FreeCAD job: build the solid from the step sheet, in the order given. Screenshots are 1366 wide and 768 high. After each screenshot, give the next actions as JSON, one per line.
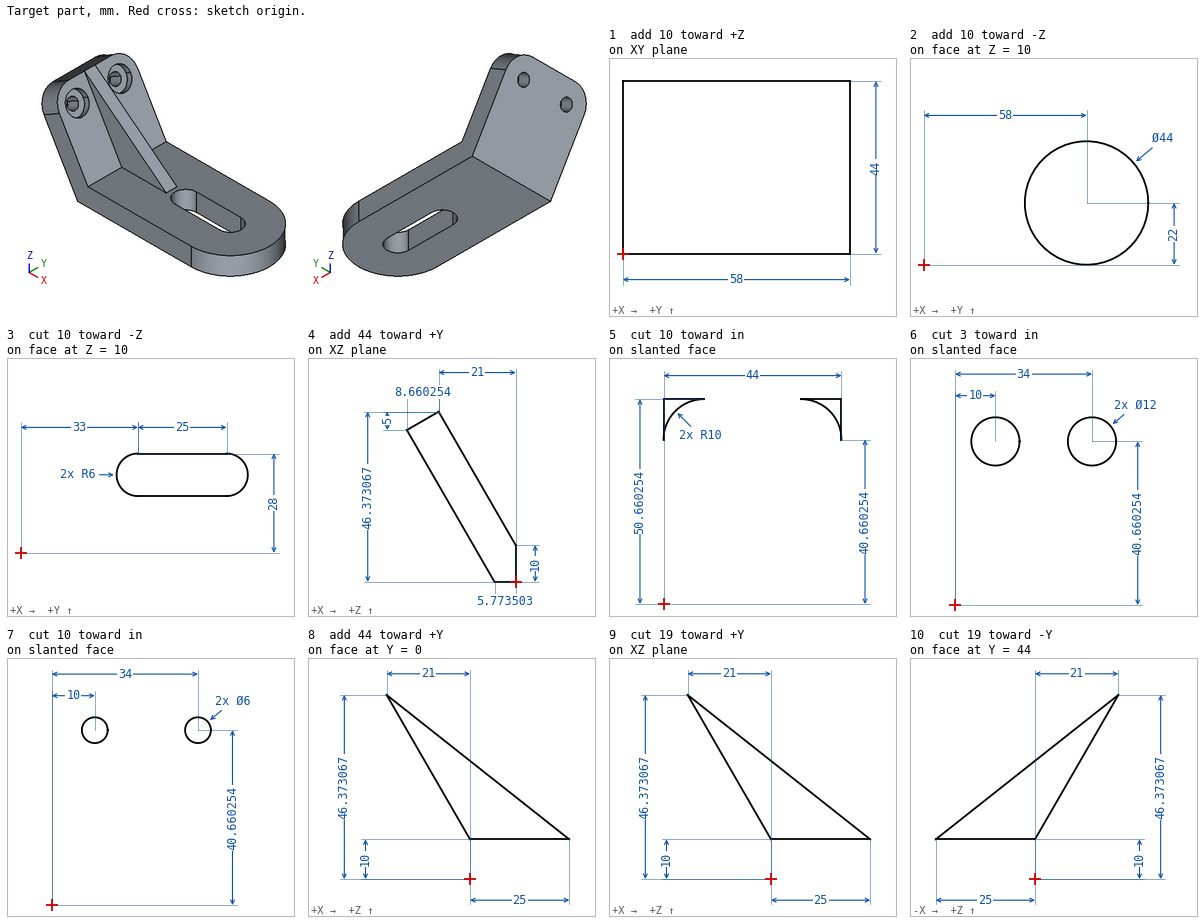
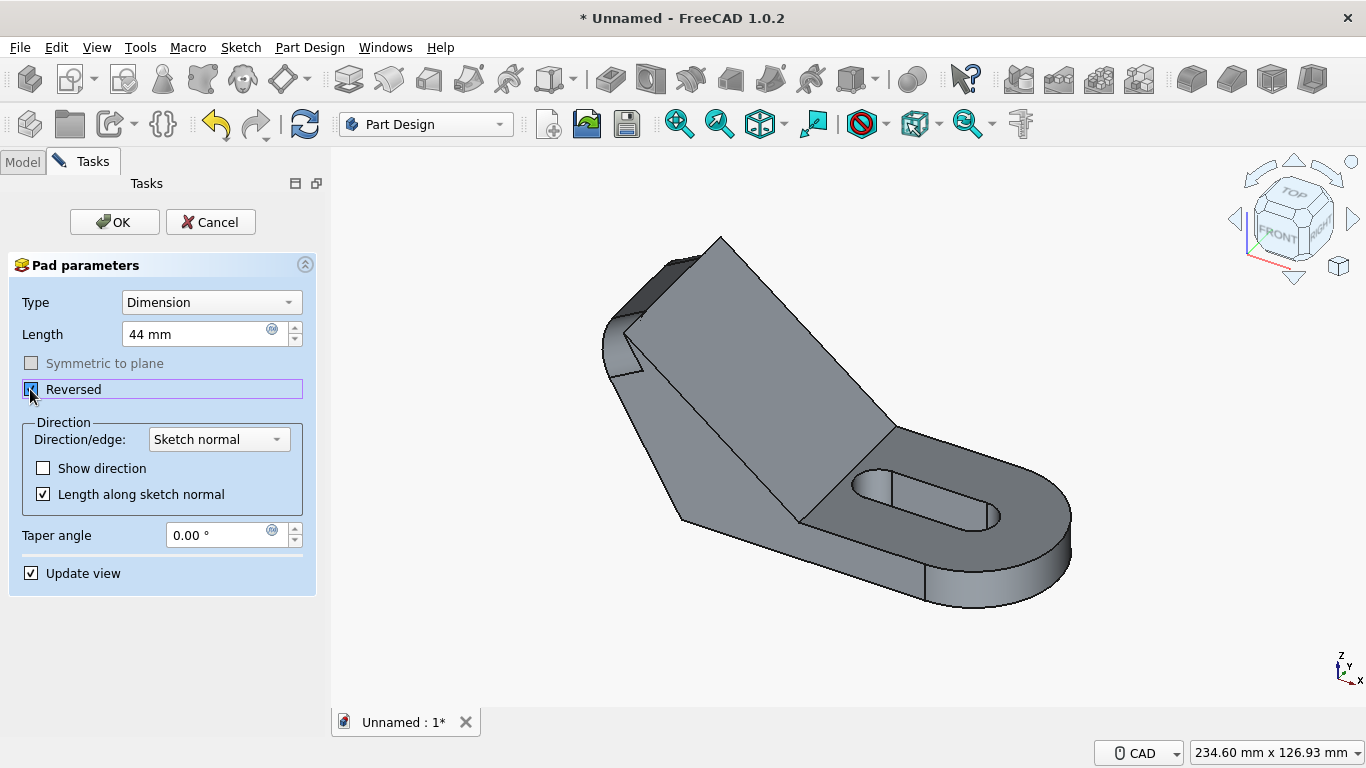
{"action": "left_click", "coordinate": [115, 222]}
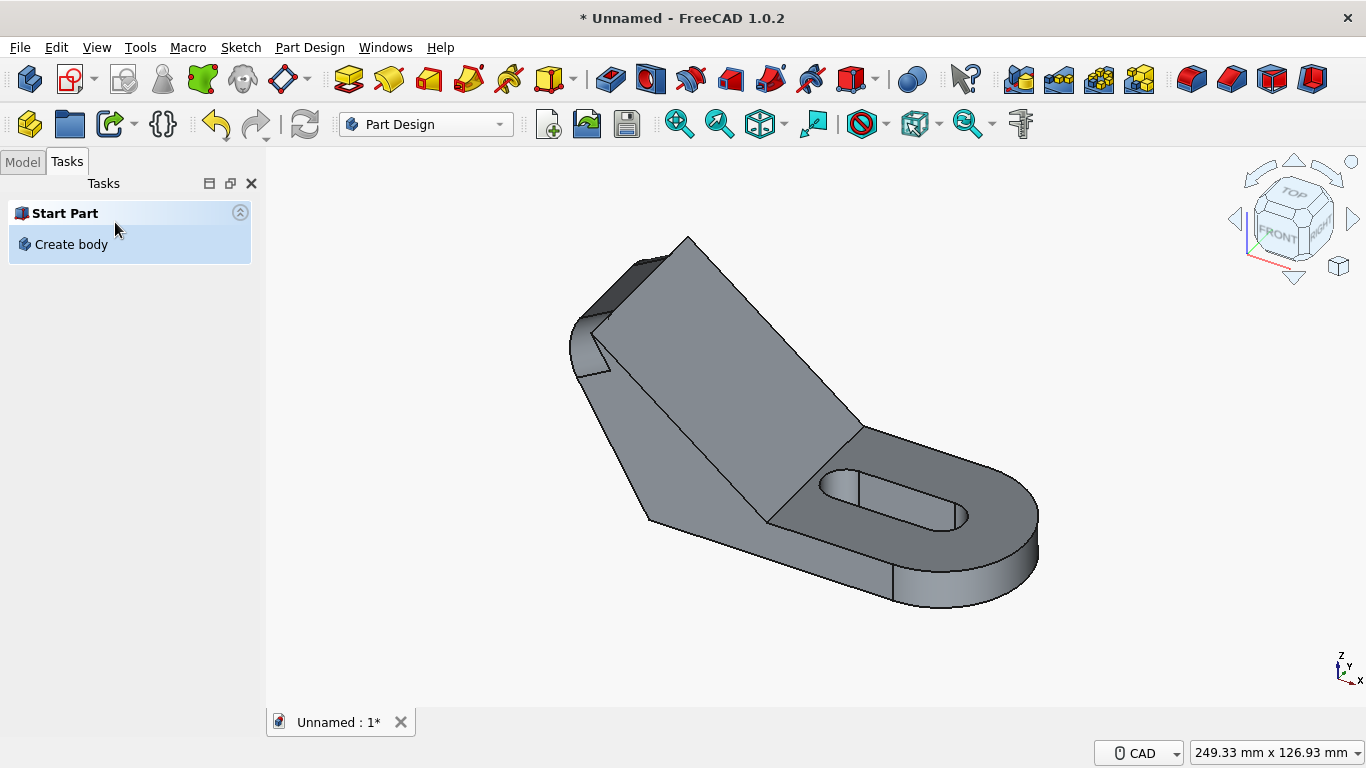
{"action": "left_click", "coordinate": [70, 80]}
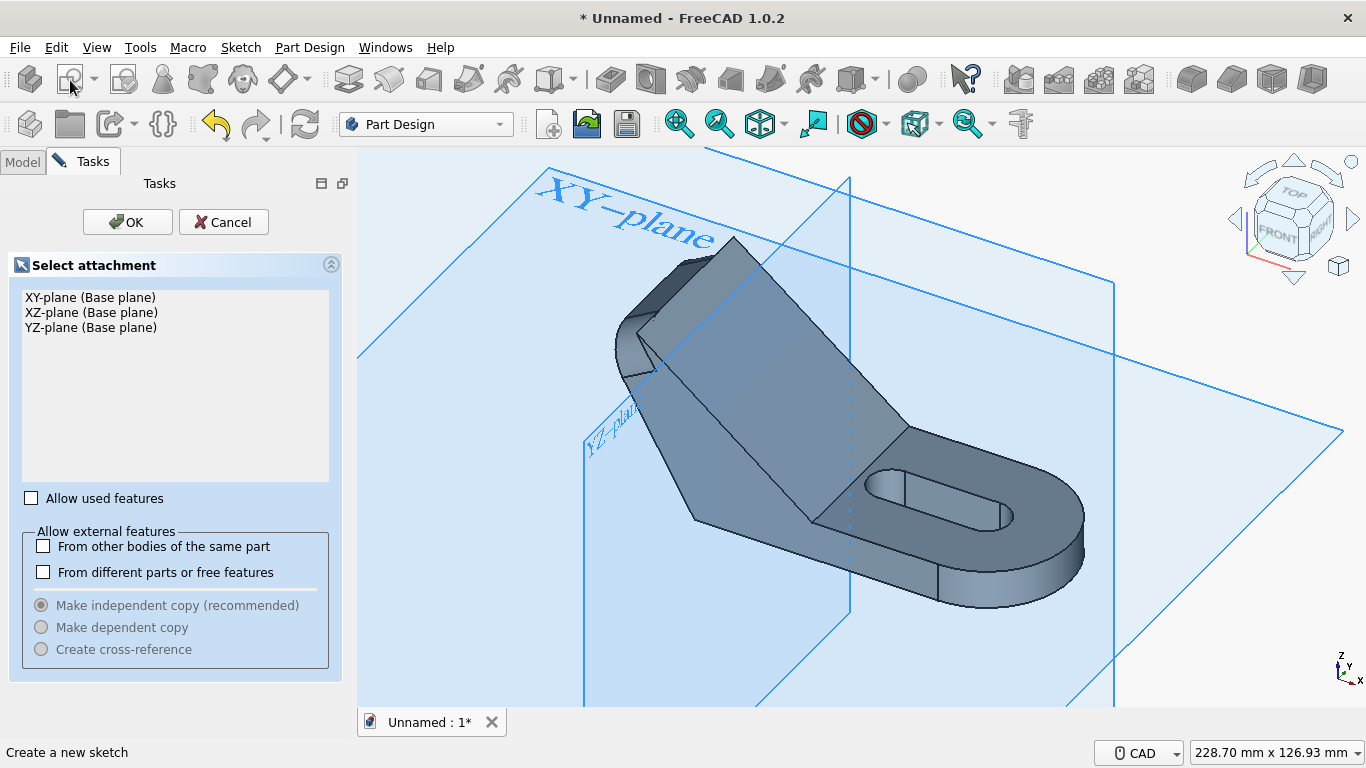
{"action": "left_click", "coordinate": [82, 312]}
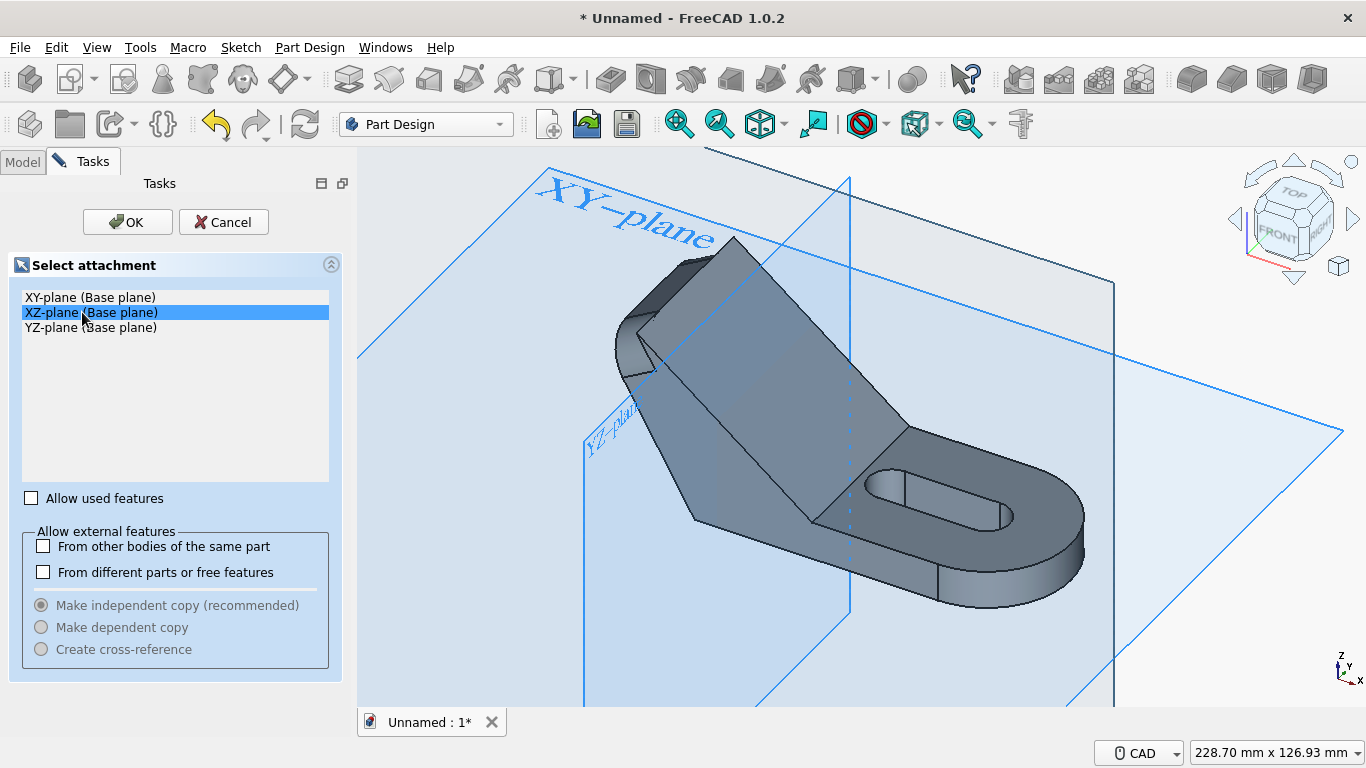
{"action": "left_click", "coordinate": [128, 222]}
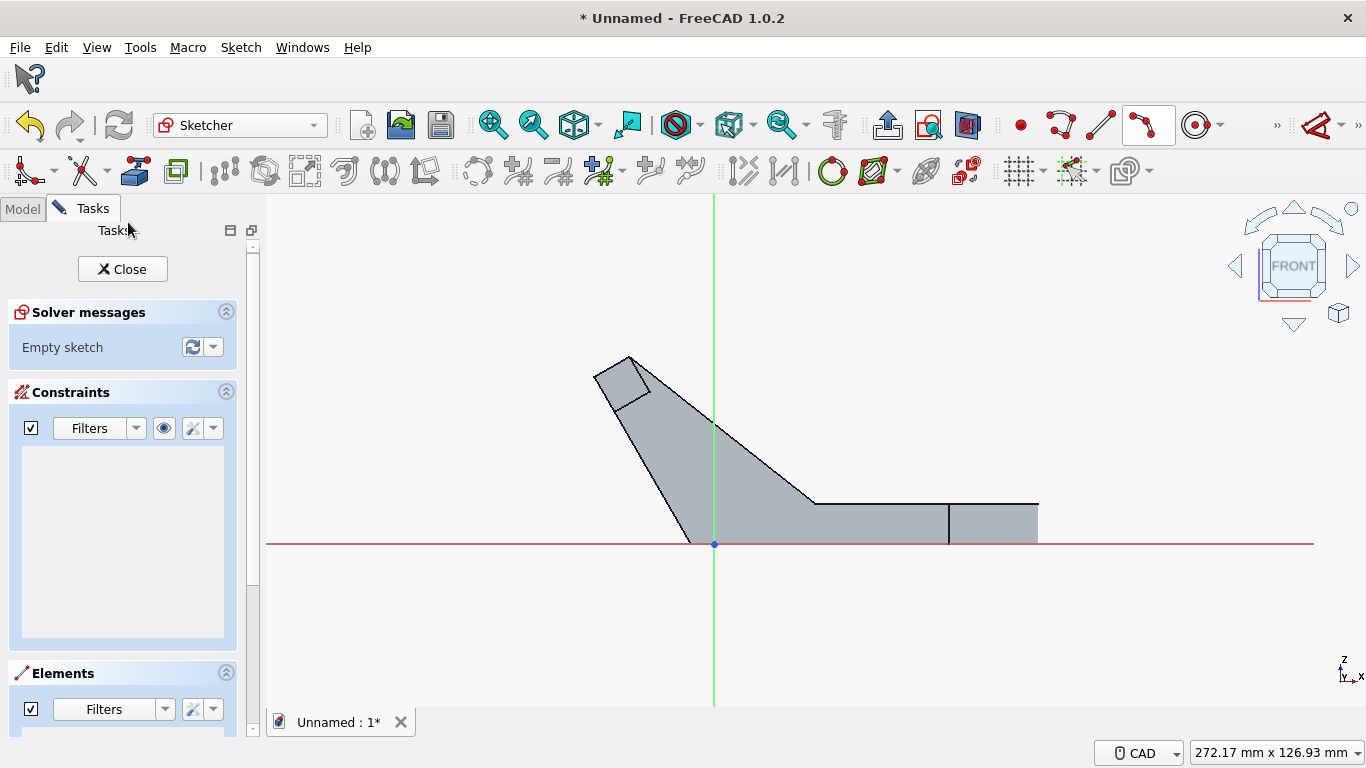
{"action": "scroll", "coordinate": [692, 451], "scroll_direction": "up", "scroll_amount": 3}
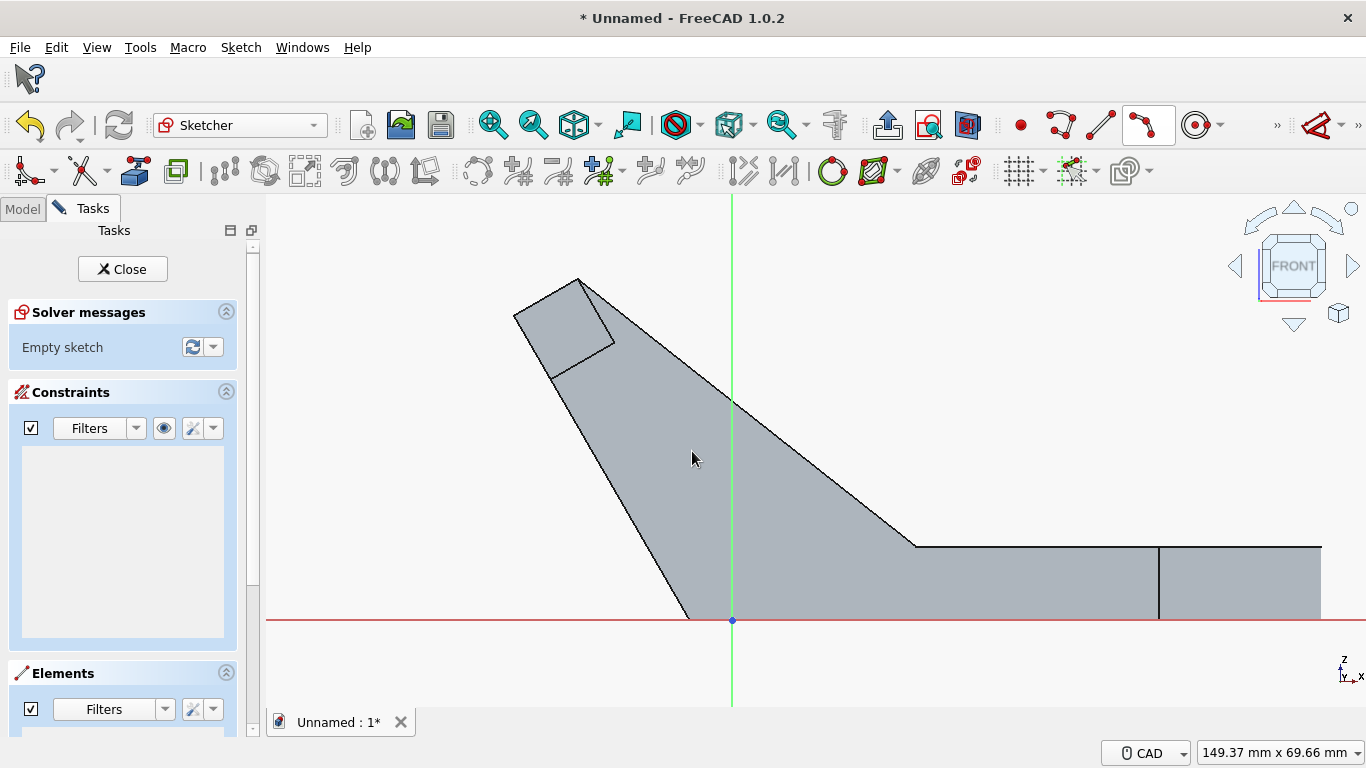
{"action": "left_click", "coordinate": [1062, 126]}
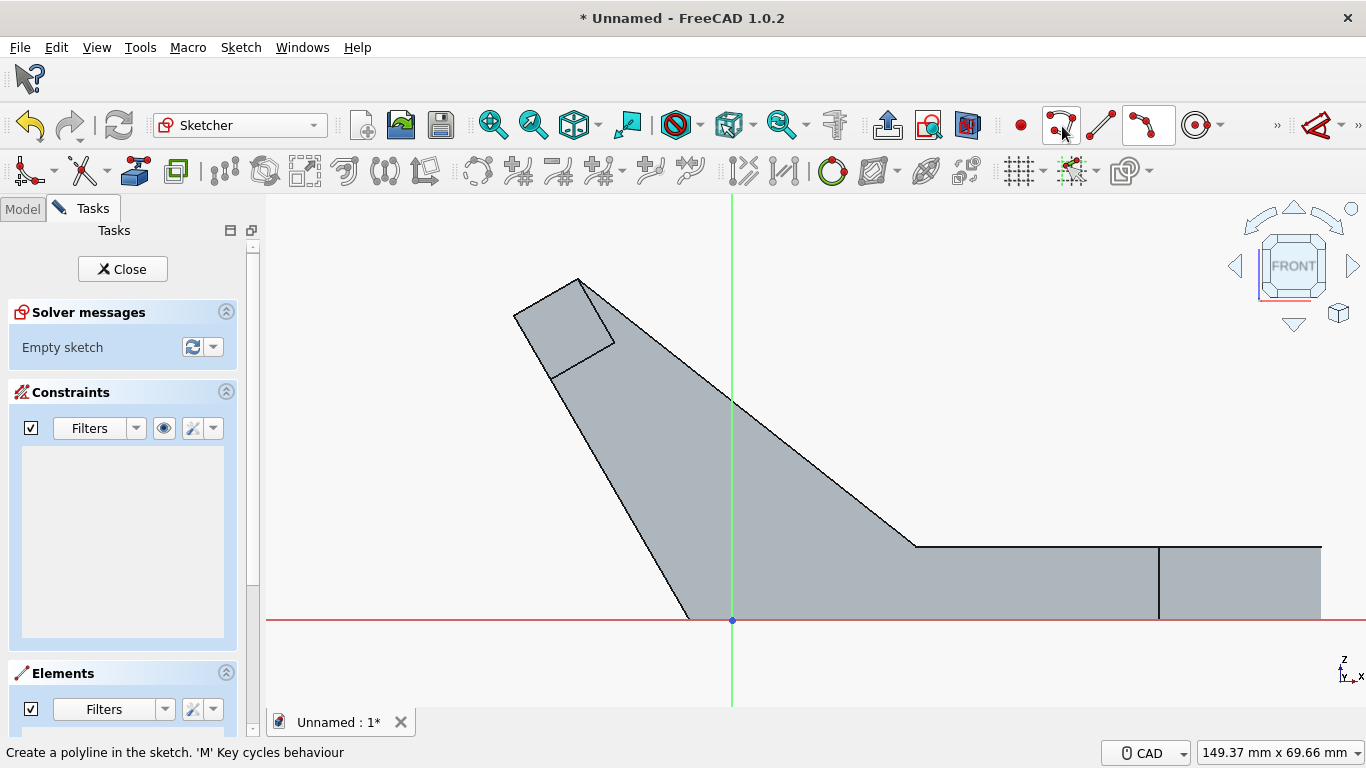
{"action": "left_click", "coordinate": [732, 547]}
{"action": "left_click", "coordinate": [916, 547]}
{"action": "left_click", "coordinate": [578, 279]}
{"action": "left_click", "coordinate": [732, 548]}
{"action": "key", "text": "Escape"}
{"action": "key", "text": "Escape"}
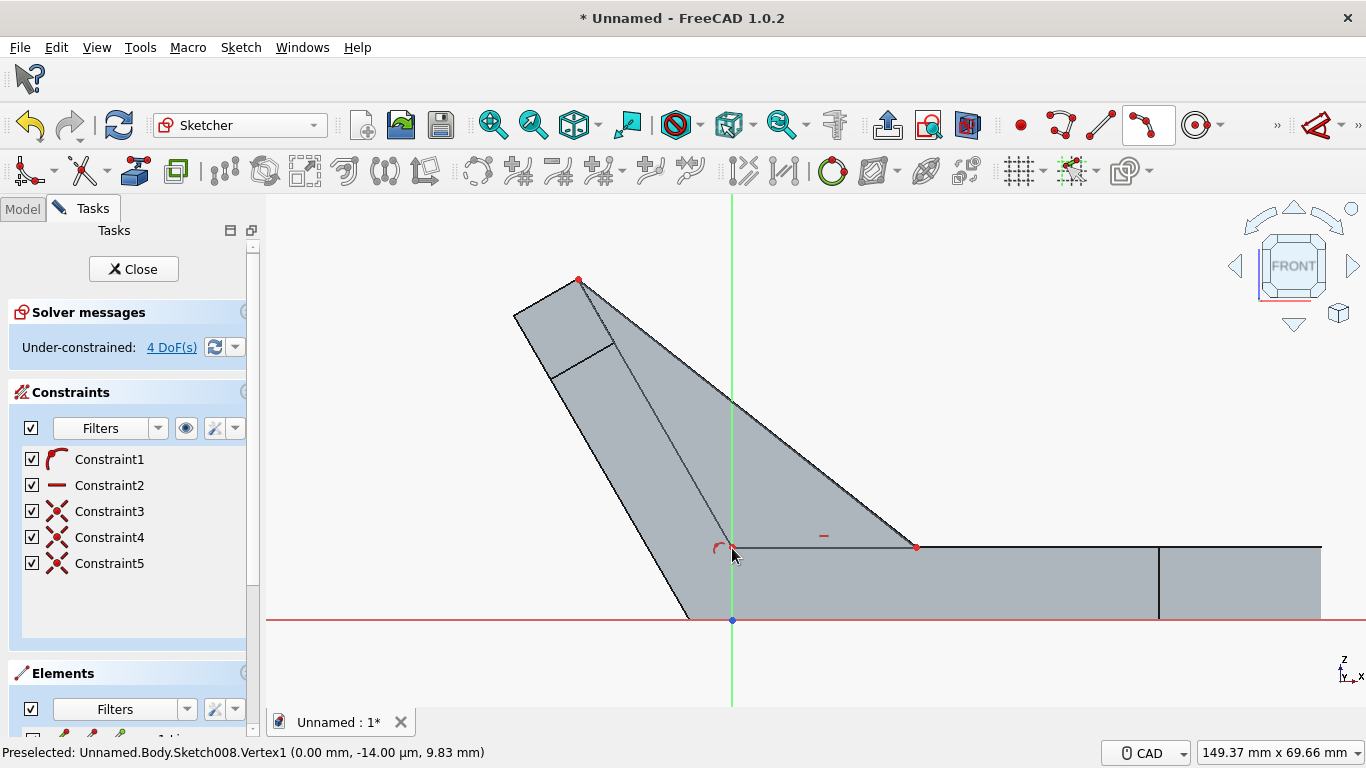
{"action": "key", "text": "d"}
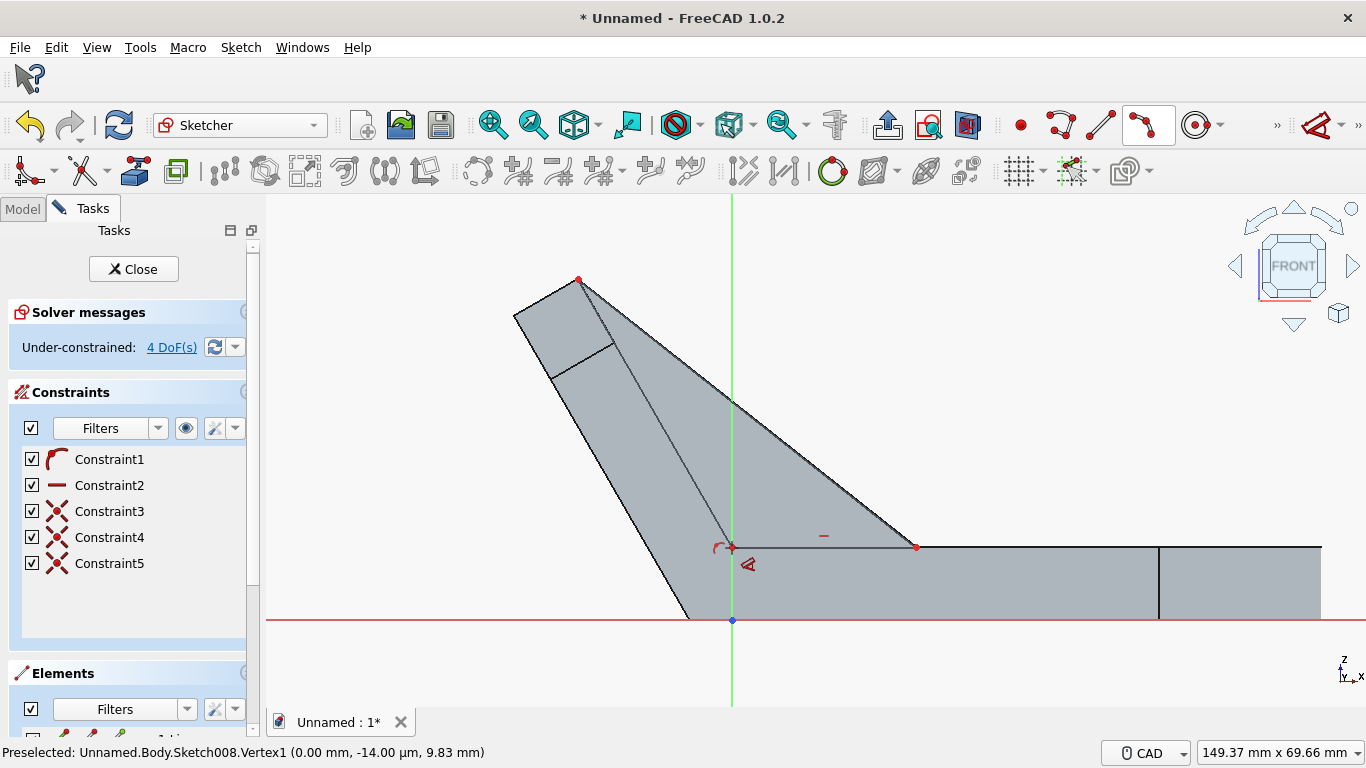
{"action": "left_click", "coordinate": [787, 548]}
{"action": "left_click", "coordinate": [824, 582]}